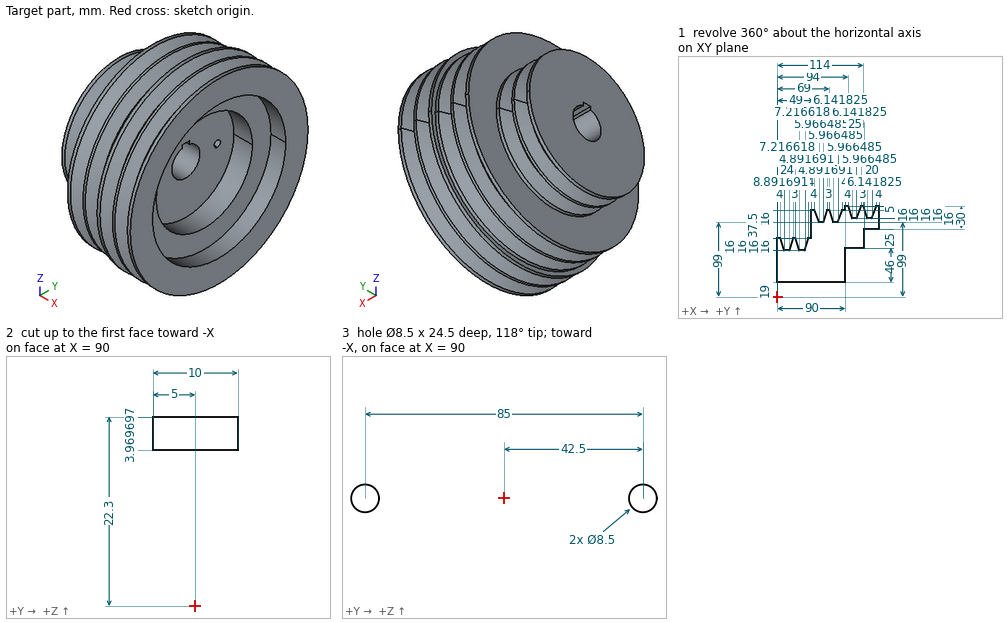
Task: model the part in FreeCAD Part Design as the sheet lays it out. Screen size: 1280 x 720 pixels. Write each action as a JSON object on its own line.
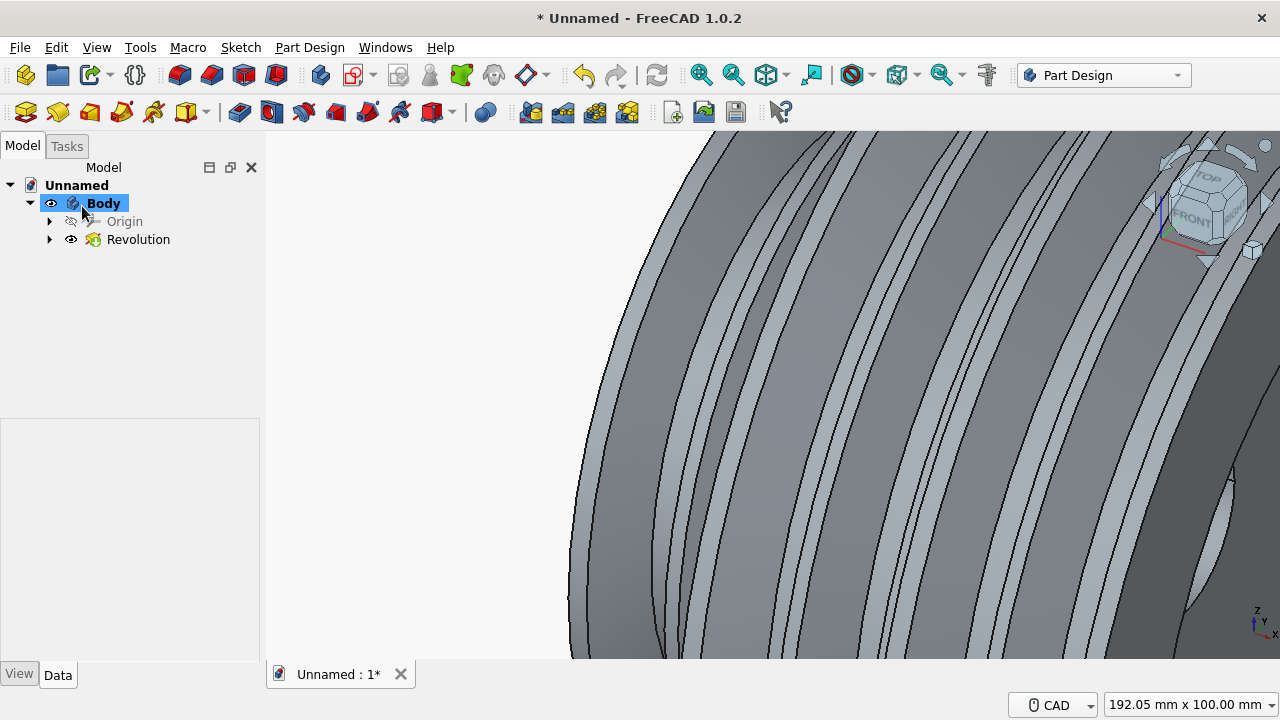
{"action": "key", "text": "v f"}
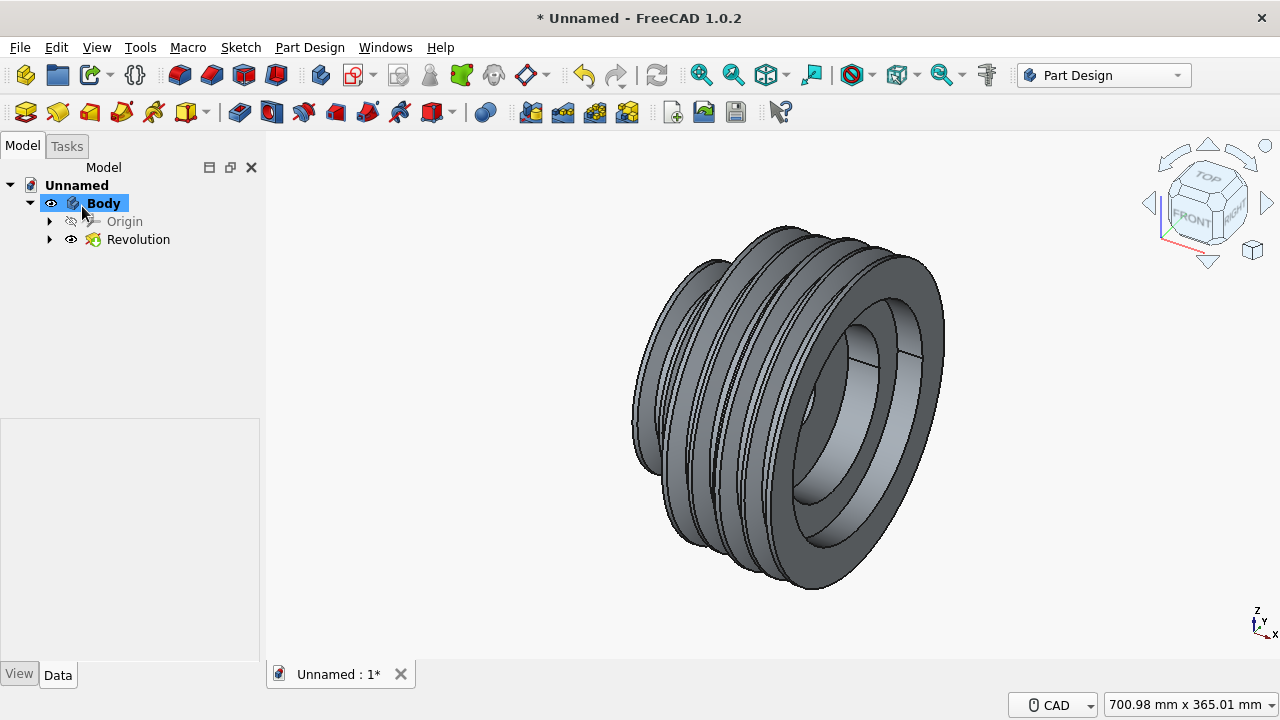
{"action": "left_click", "coordinate": [828, 399]}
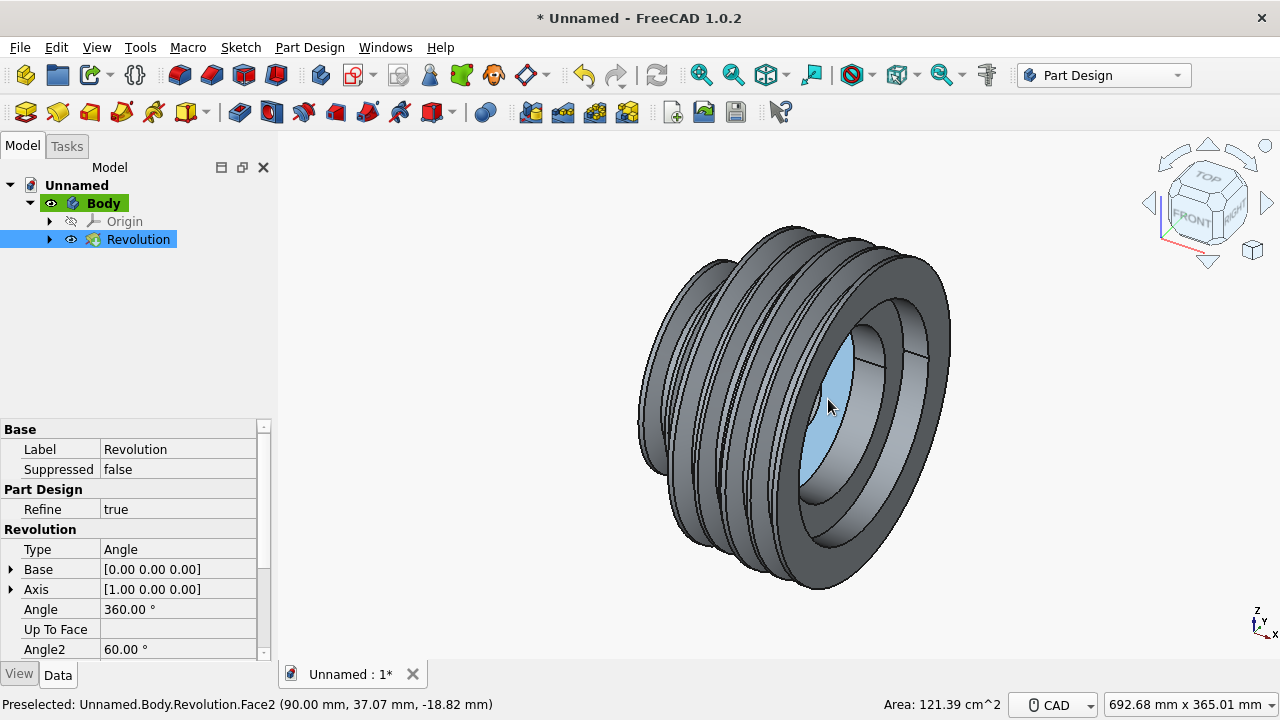
{"action": "left_click", "coordinate": [354, 76]}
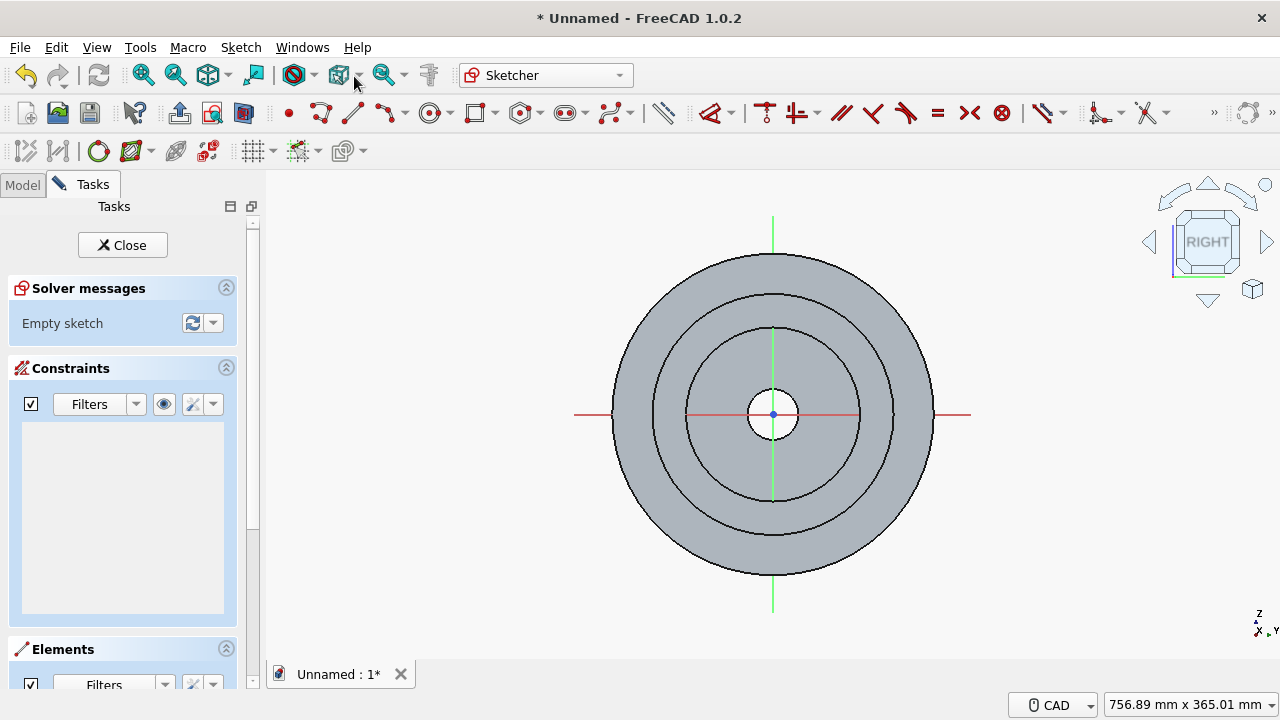
{"action": "scroll", "coordinate": [780, 398], "scroll_direction": "up", "scroll_amount": 12}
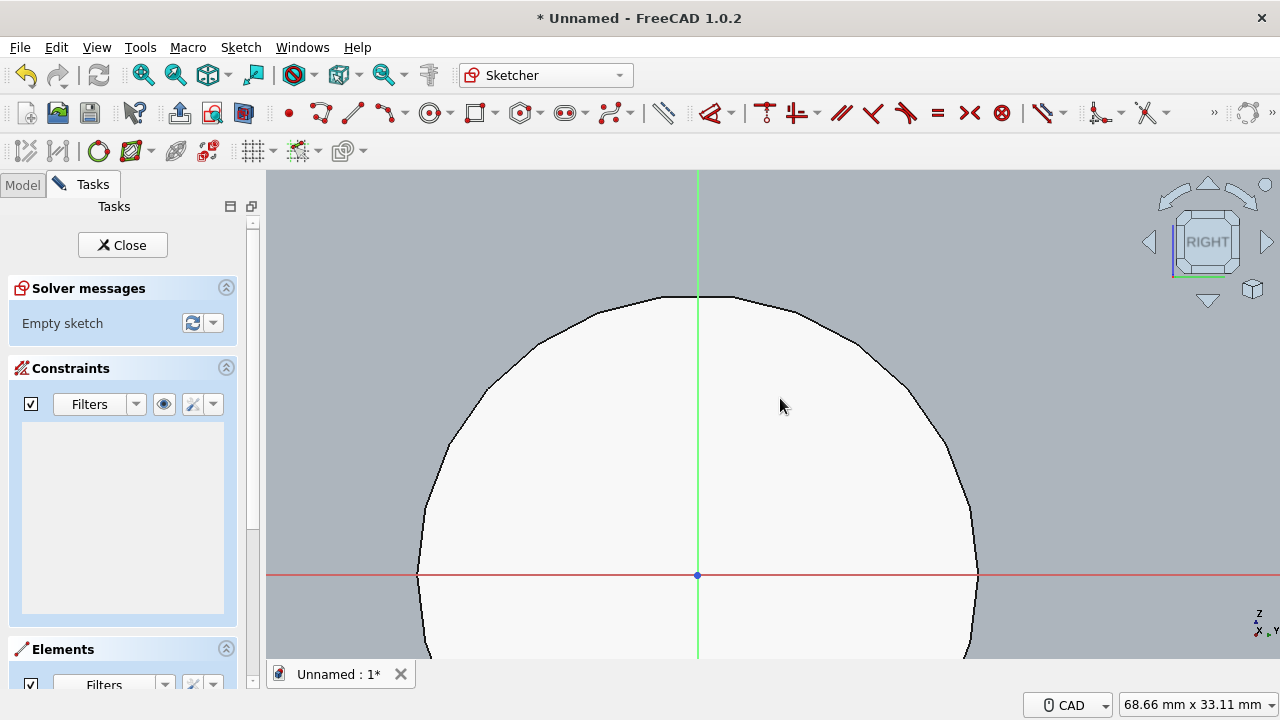
{"action": "key", "text": "g r"}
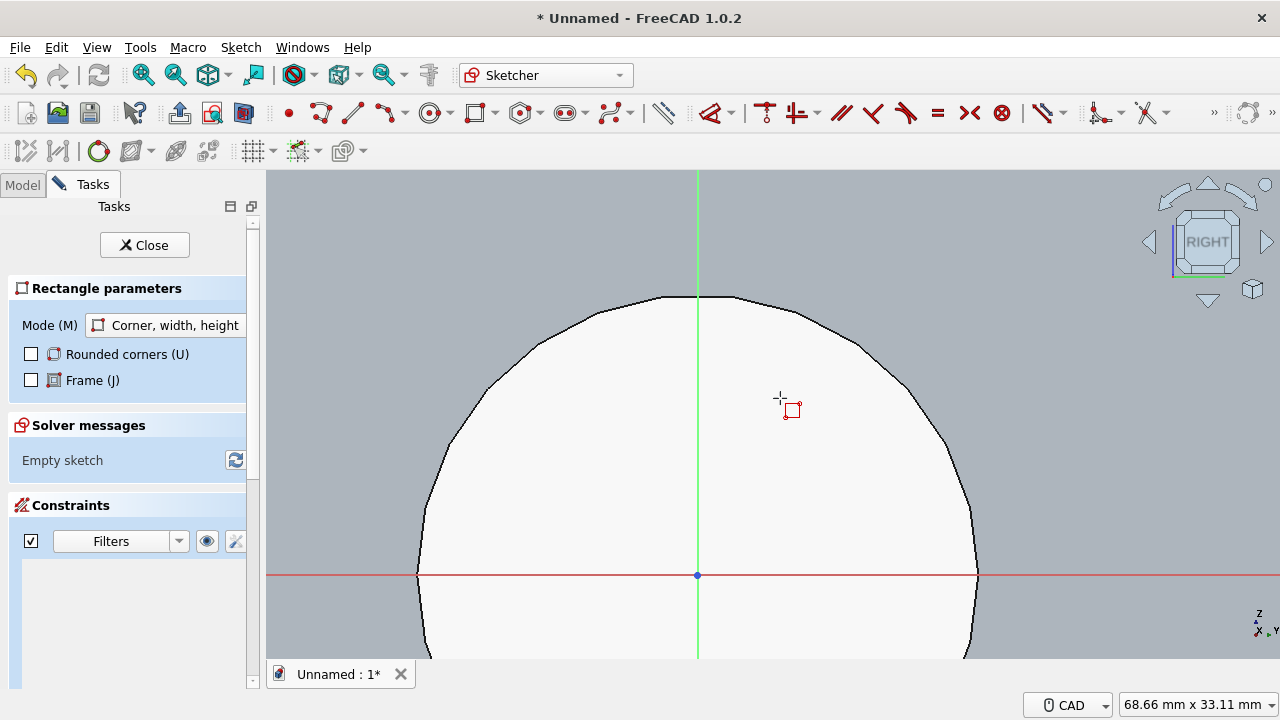
{"action": "left_click", "coordinate": [624, 246]}
{"action": "left_click", "coordinate": [772, 305]}
{"action": "key", "text": "Escape"}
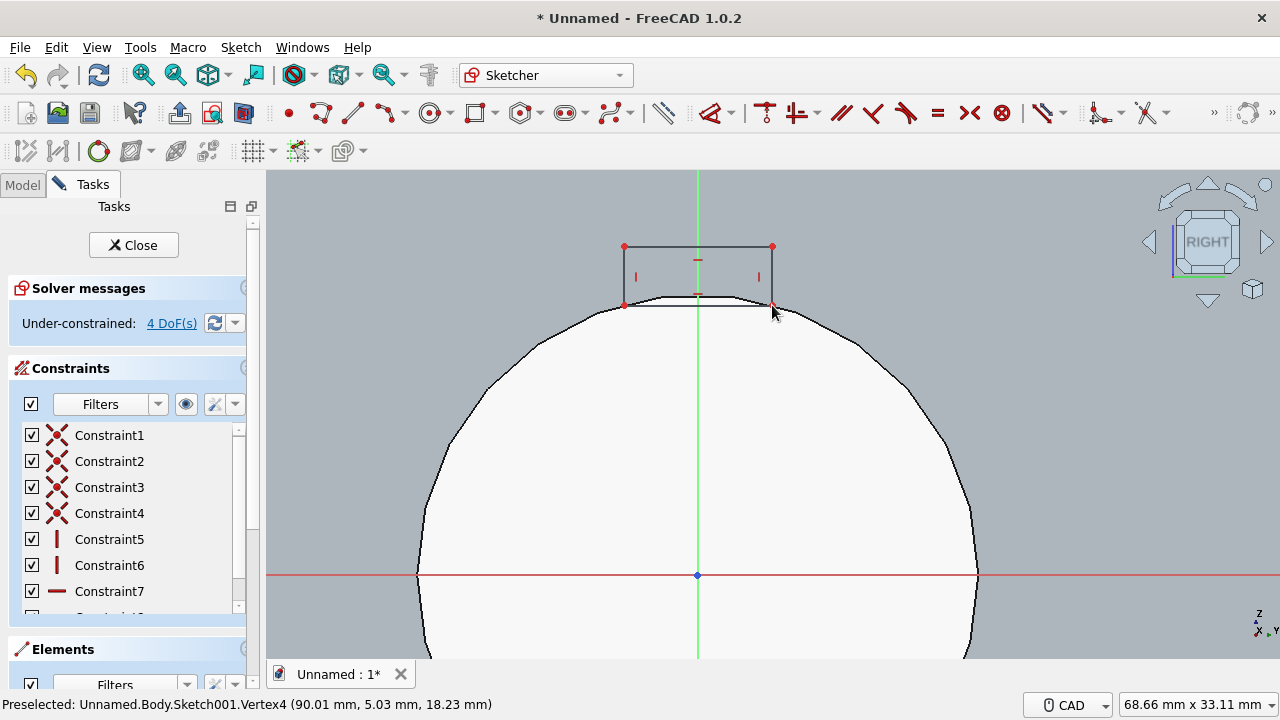
{"action": "key", "text": "d"}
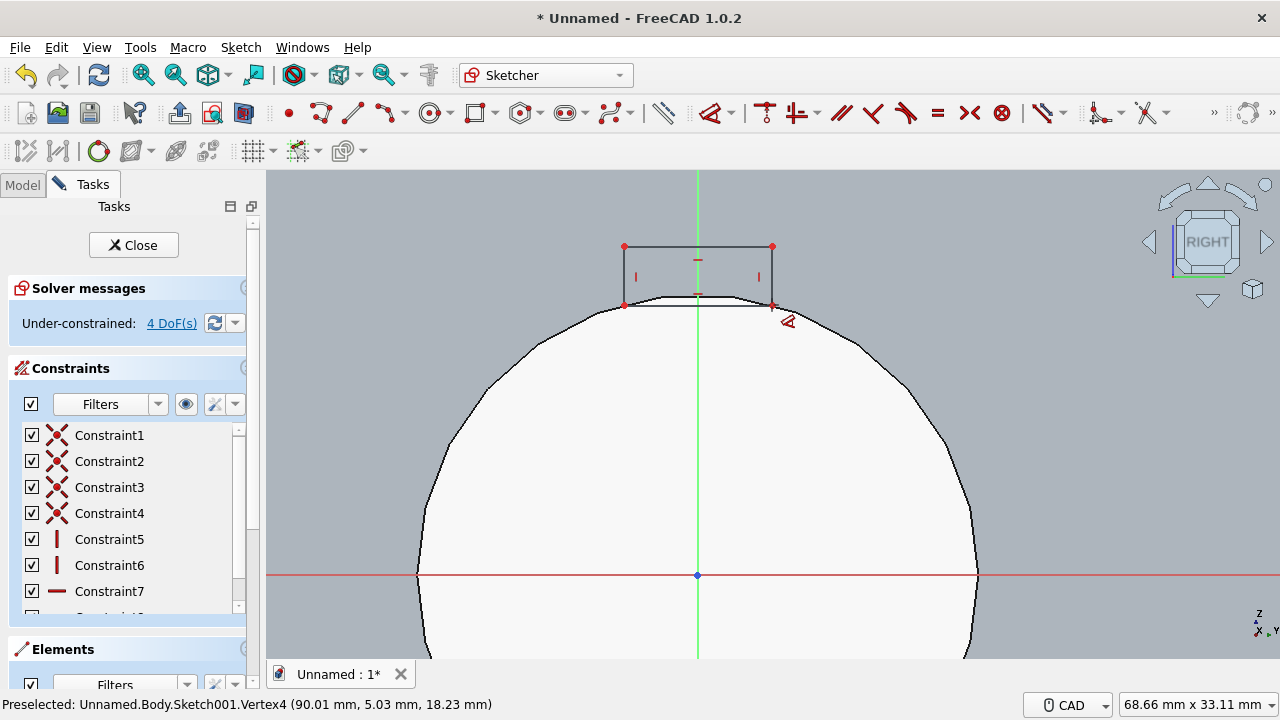
{"action": "left_click", "coordinate": [668, 306]}
{"action": "left_click", "coordinate": [664, 272]}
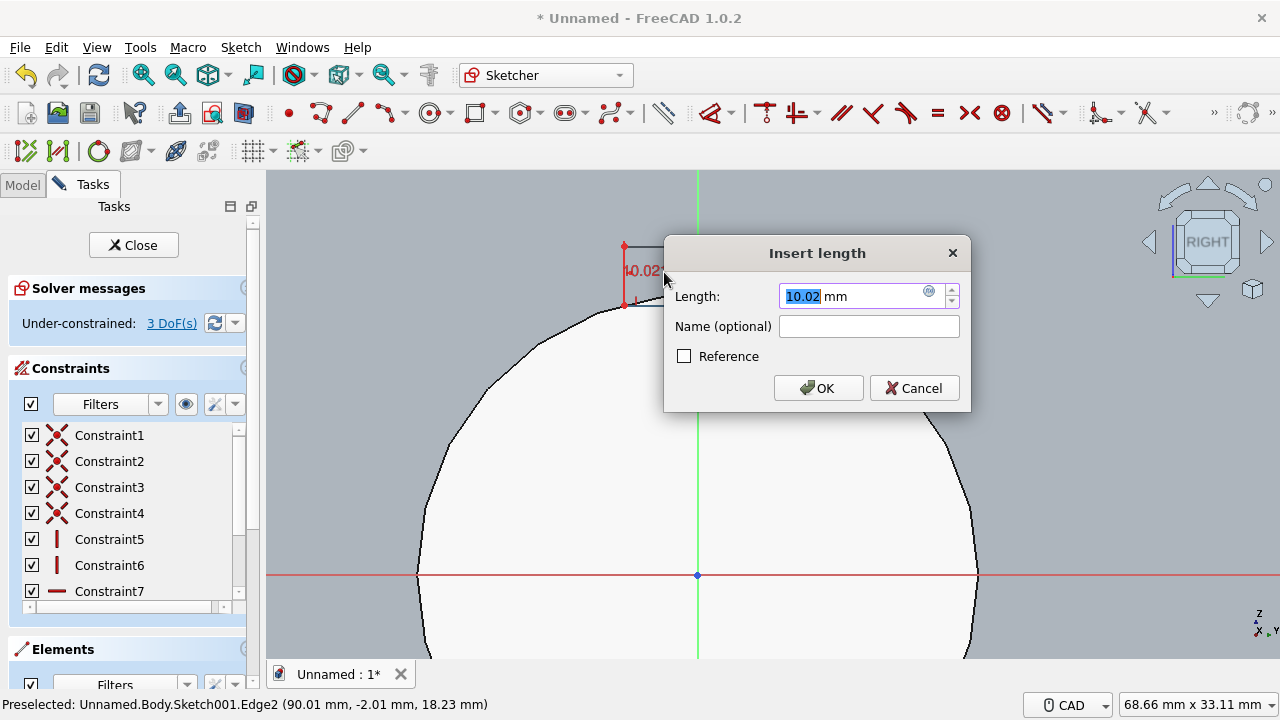
{"action": "type", "text": "10"}
{"action": "key", "text": "Return"}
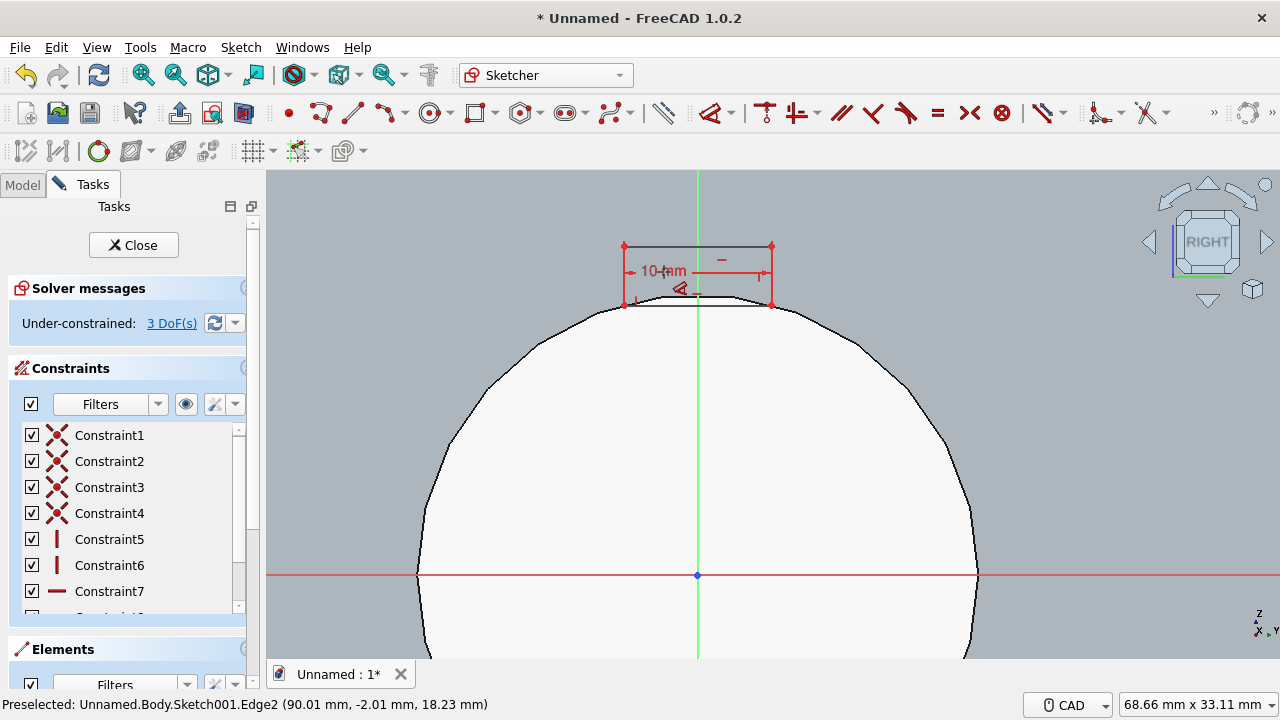
{"action": "left_click", "coordinate": [624, 247]}
{"action": "left_click", "coordinate": [661, 609]}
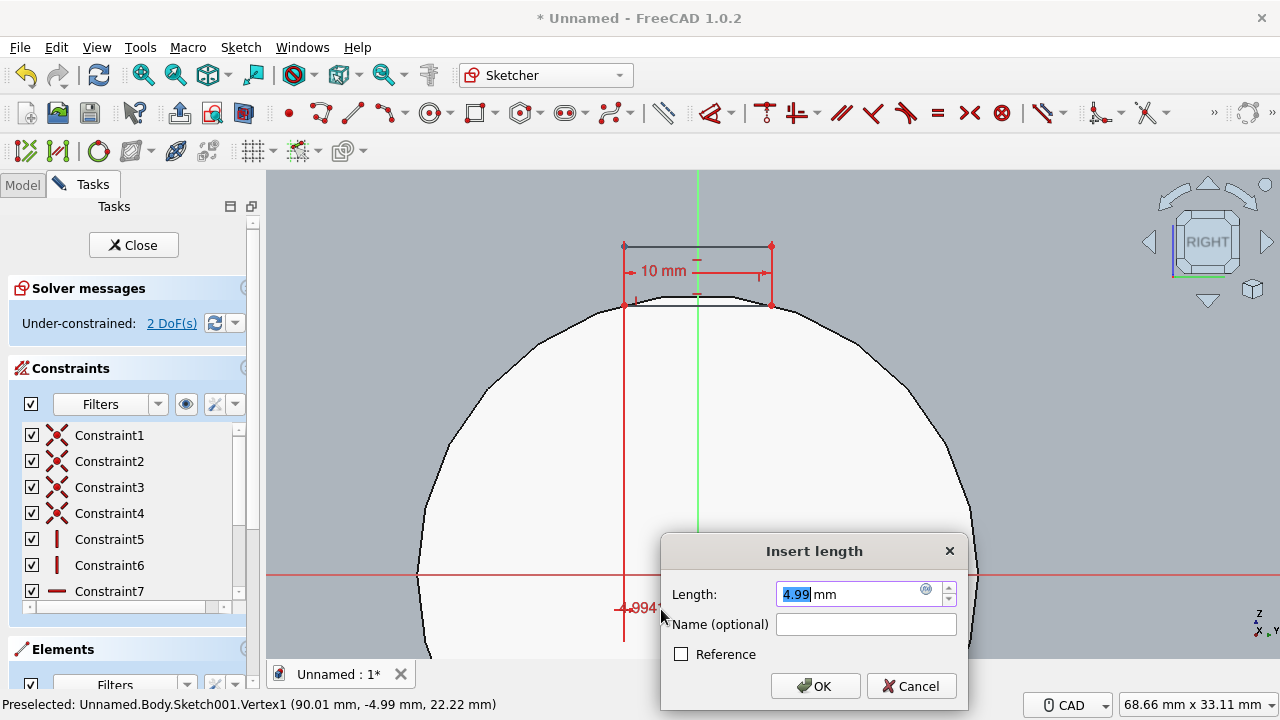
{"action": "type", "text": "5"}
{"action": "key", "text": "Return"}